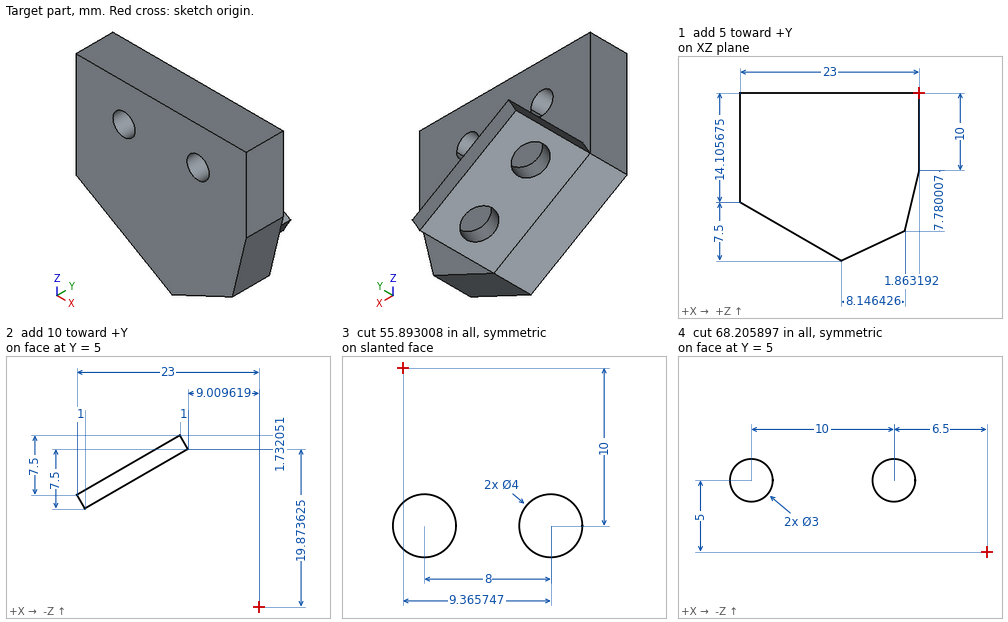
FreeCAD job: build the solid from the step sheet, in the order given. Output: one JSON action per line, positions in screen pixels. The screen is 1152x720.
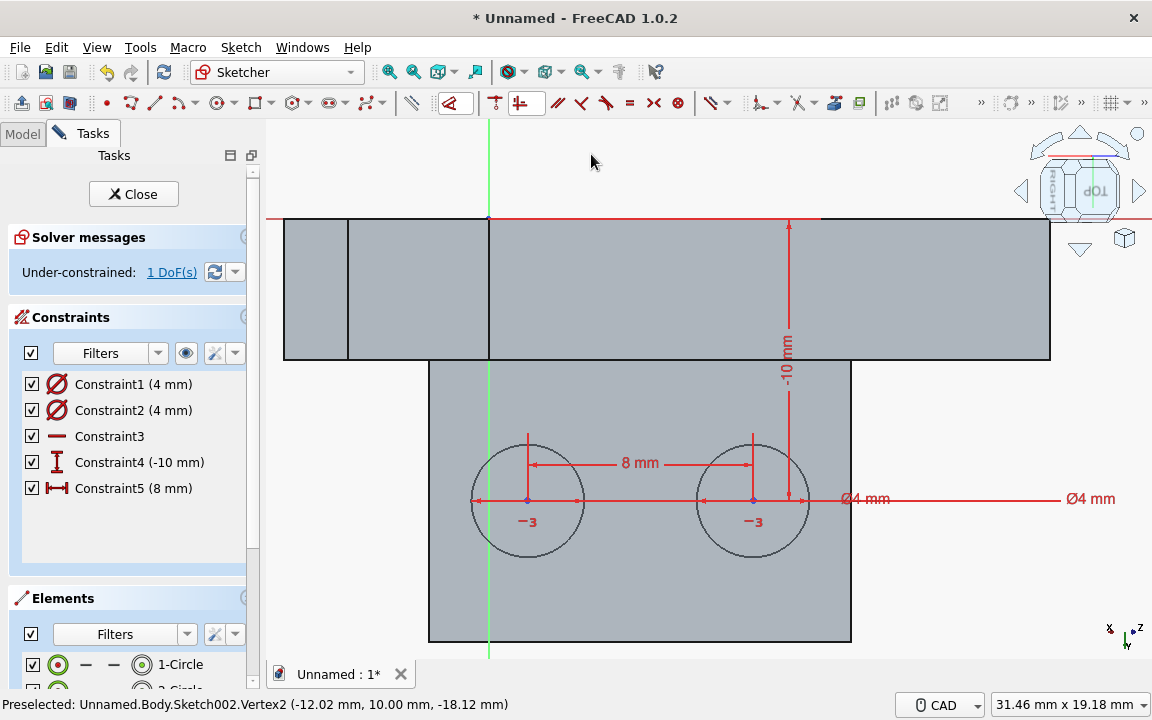
{"action": "left_click", "coordinate": [753, 501]}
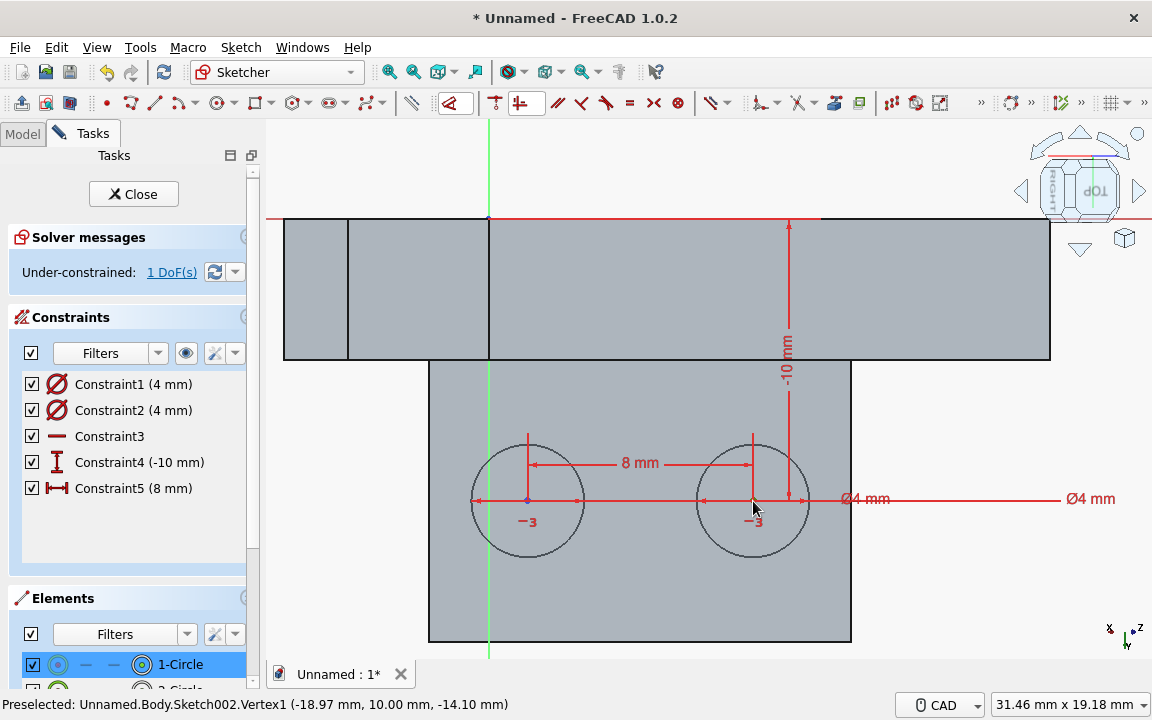
{"action": "key", "text": "l"}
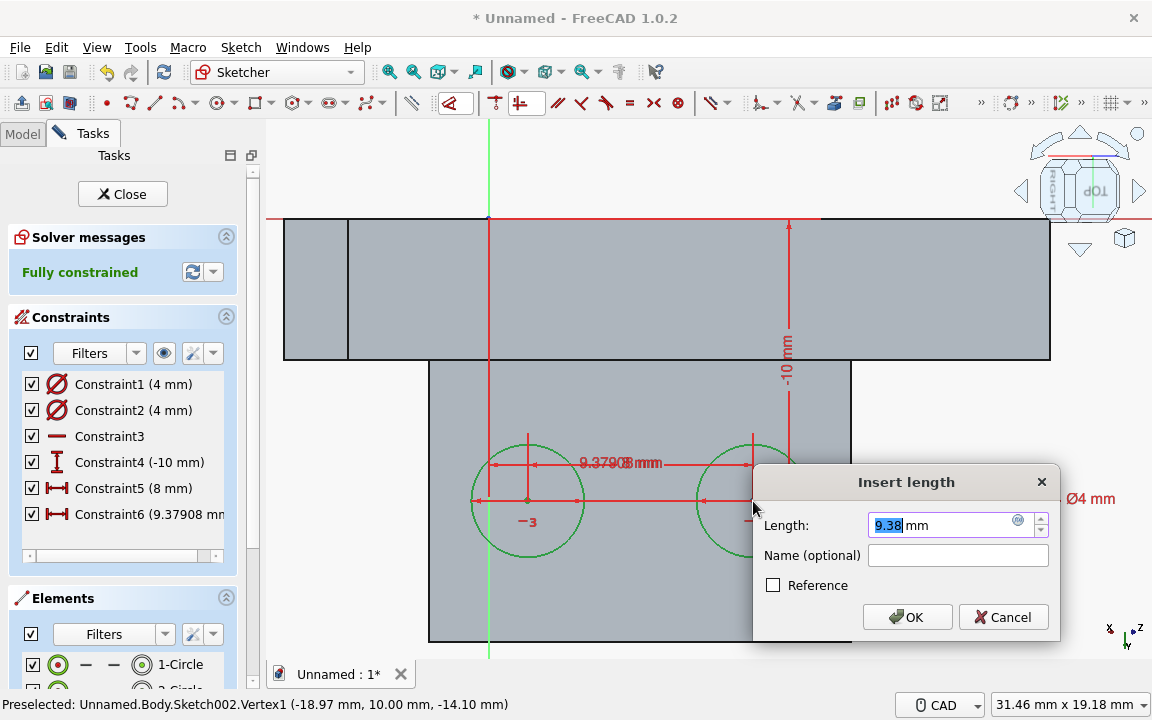
{"action": "type", "text": "9.365747"}
{"action": "key", "text": "Return"}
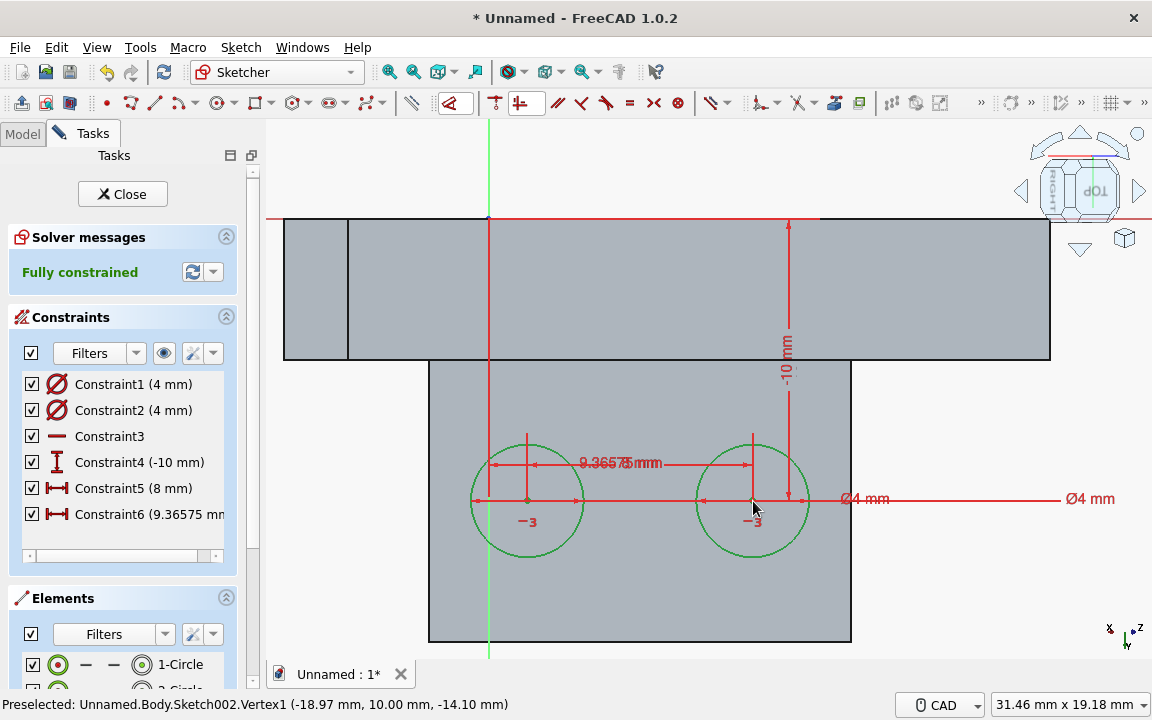
{"action": "left_click", "coordinate": [123, 194]}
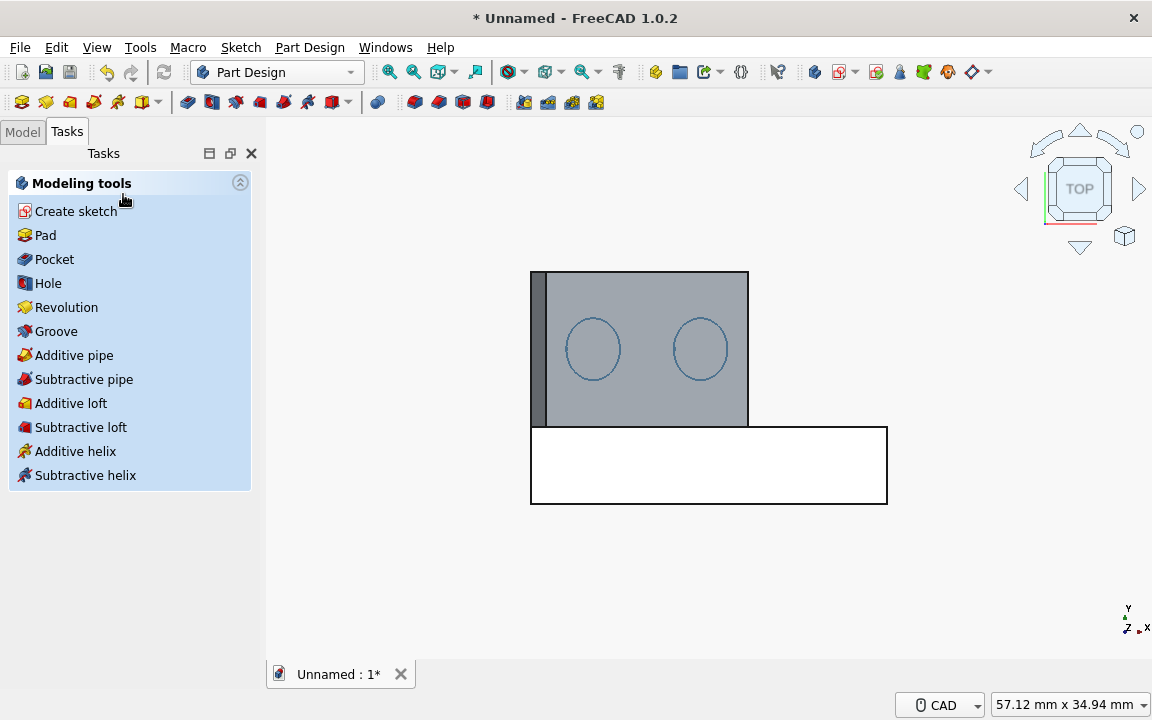
{"action": "left_click", "coordinate": [188, 102]}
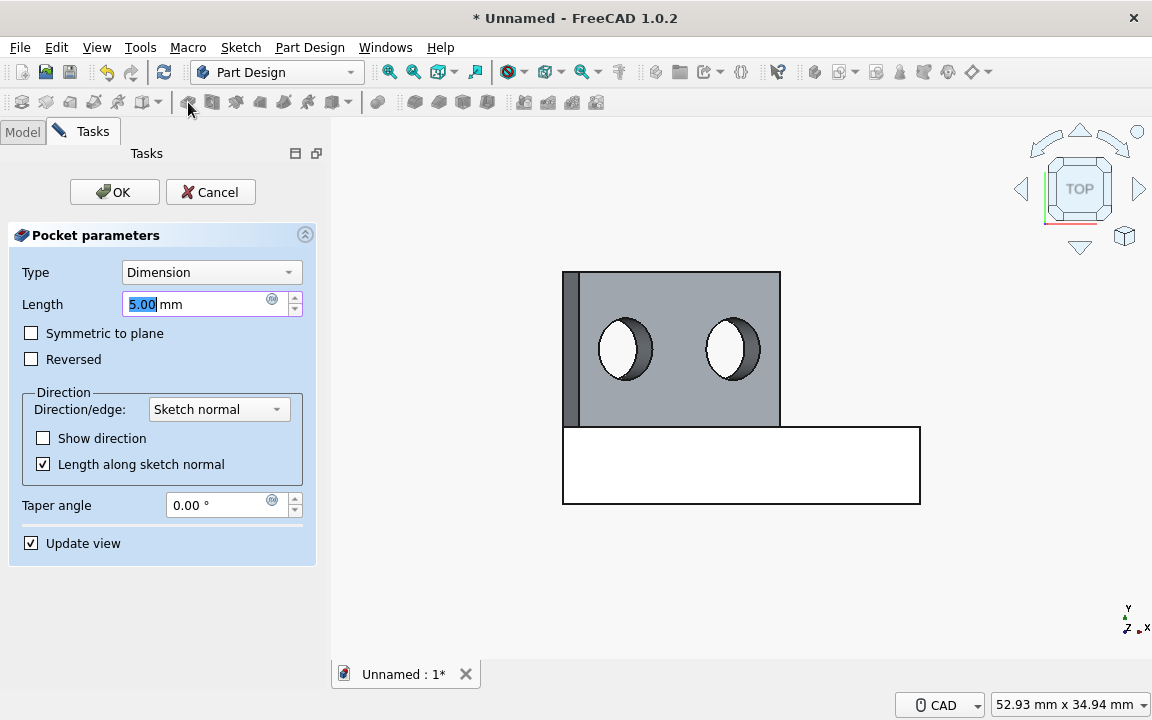
{"action": "type", "text": "55.893008"}
{"action": "key", "text": "Tab"}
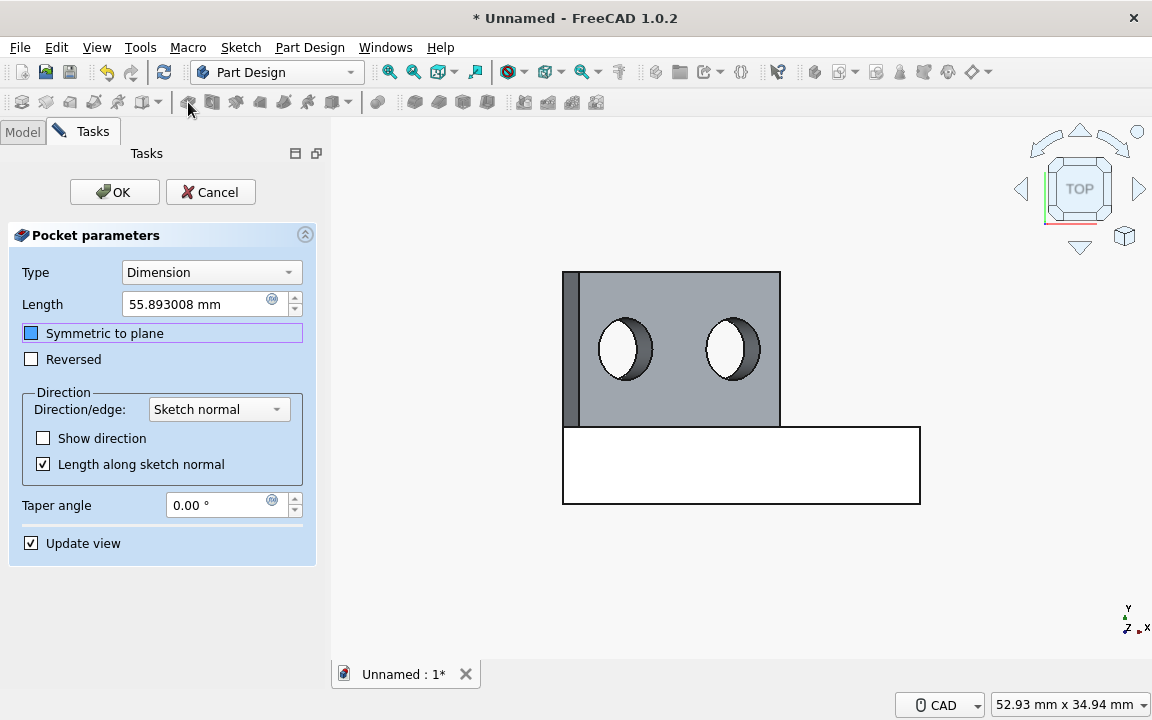
{"action": "left_click", "coordinate": [30, 333]}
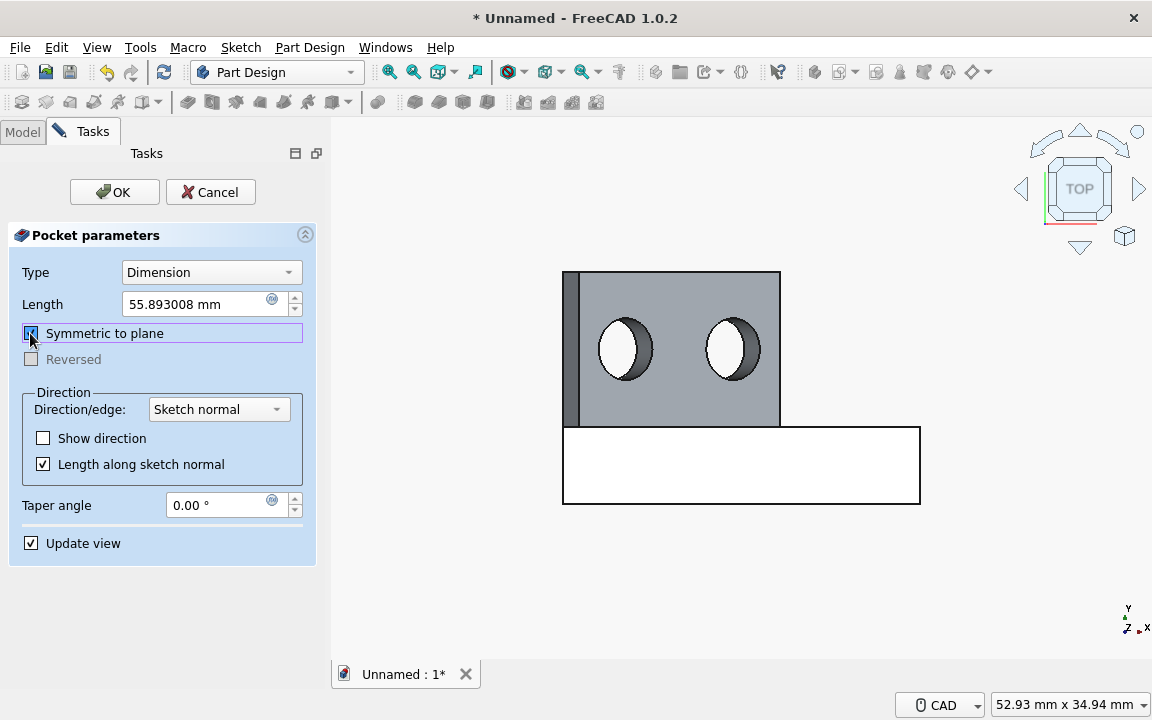
{"action": "left_click", "coordinate": [115, 192]}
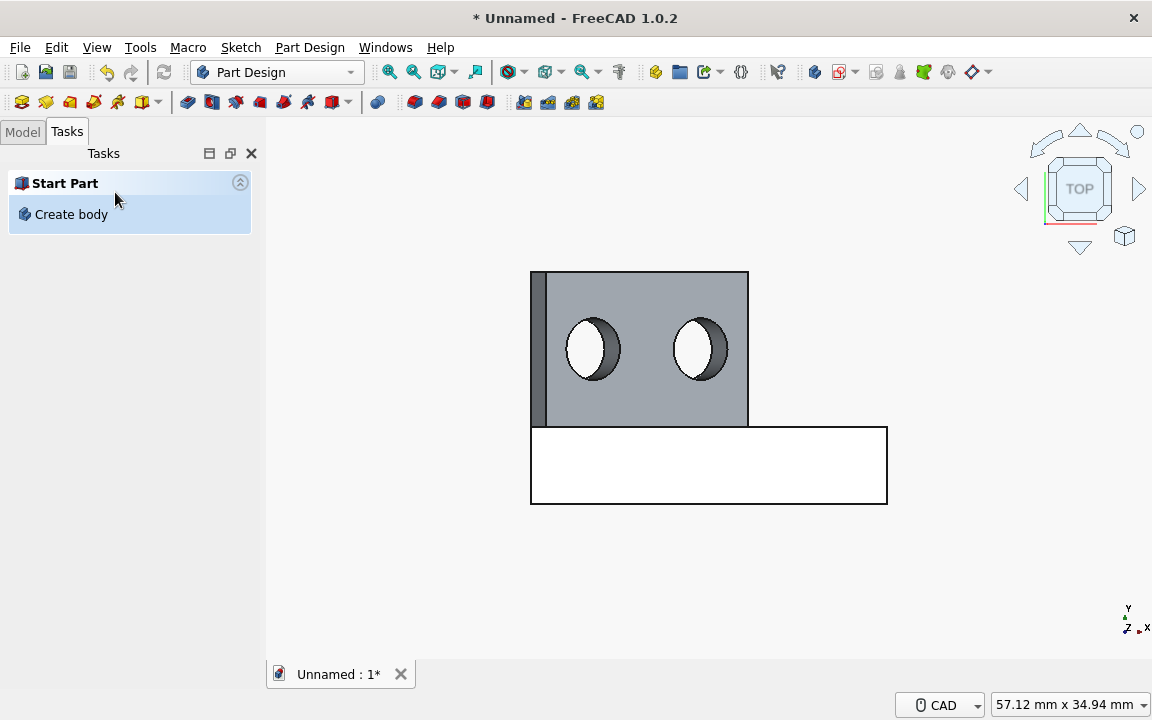
{"action": "left_click", "coordinate": [390, 72]}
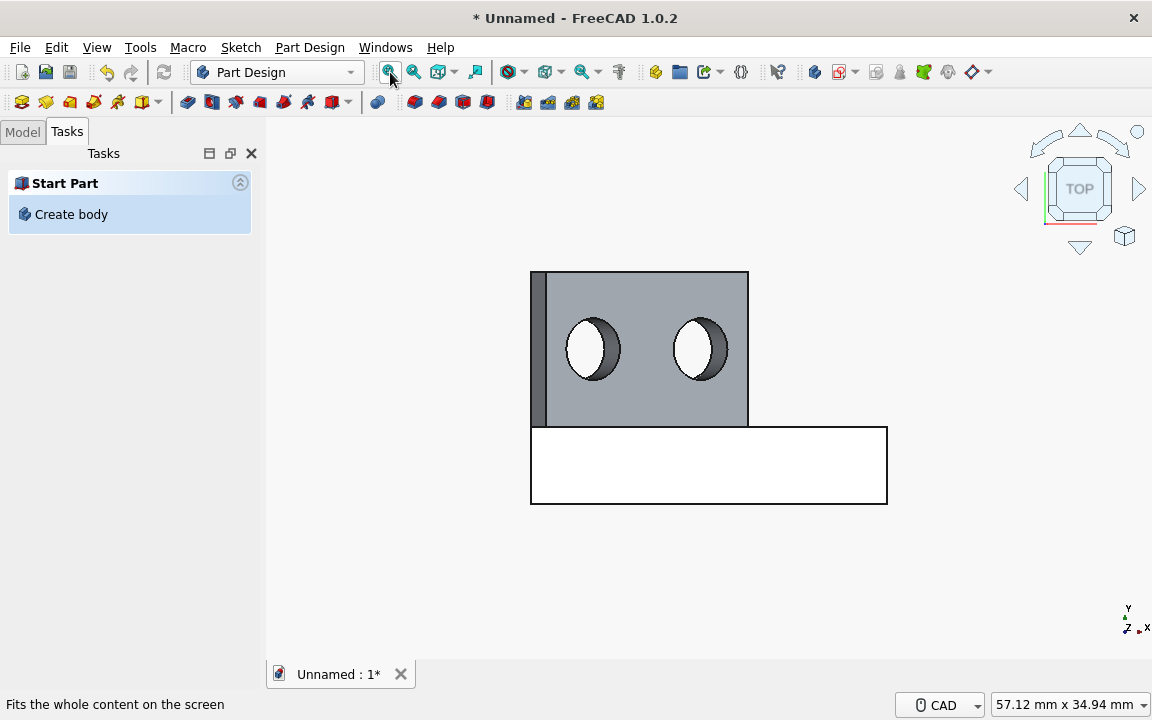
{"action": "key", "text": "4"}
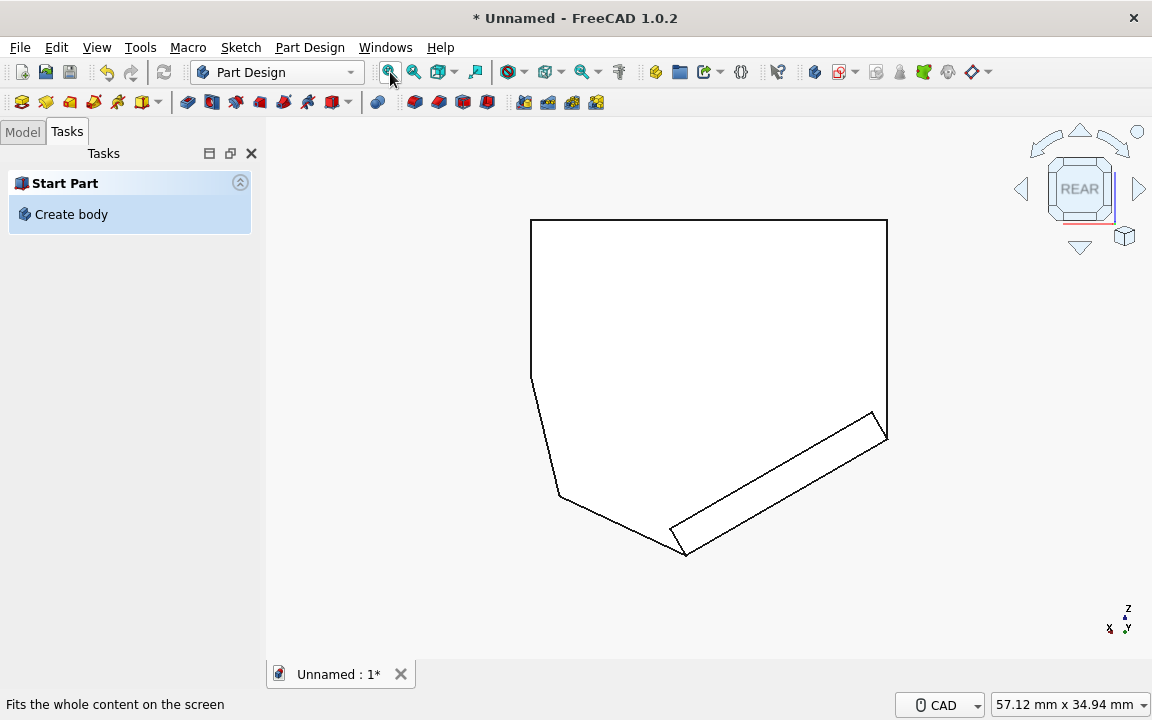
{"action": "left_click", "coordinate": [658, 387]}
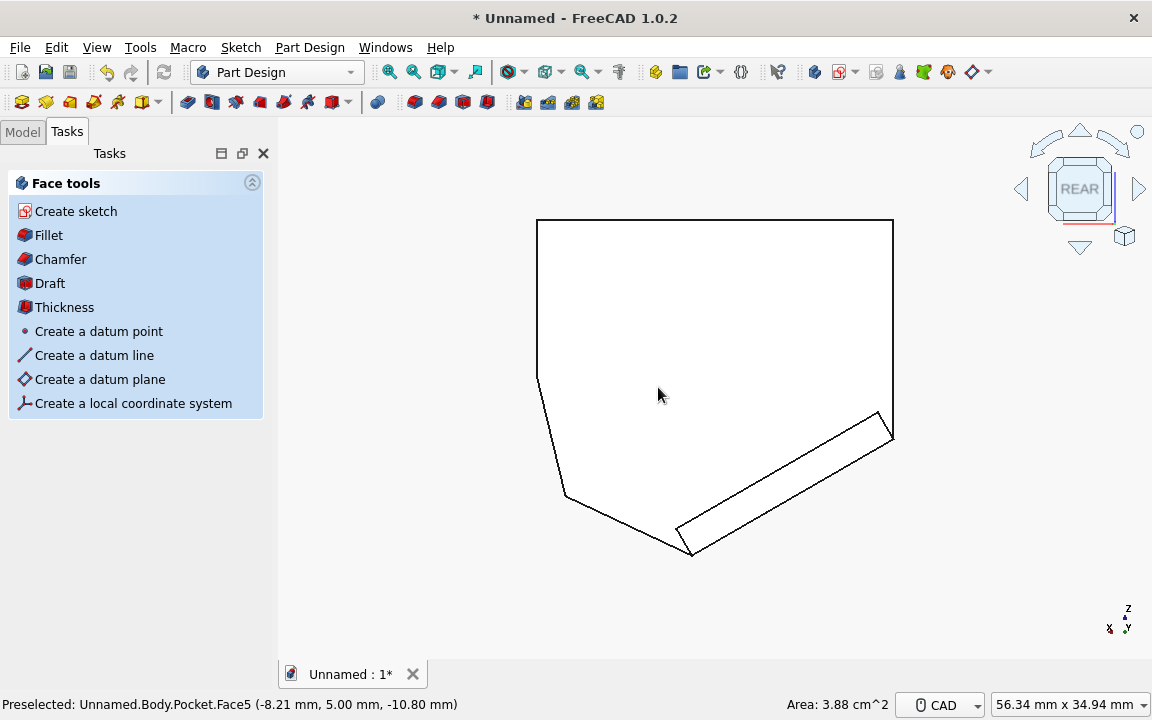
{"action": "left_click", "coordinate": [840, 72]}